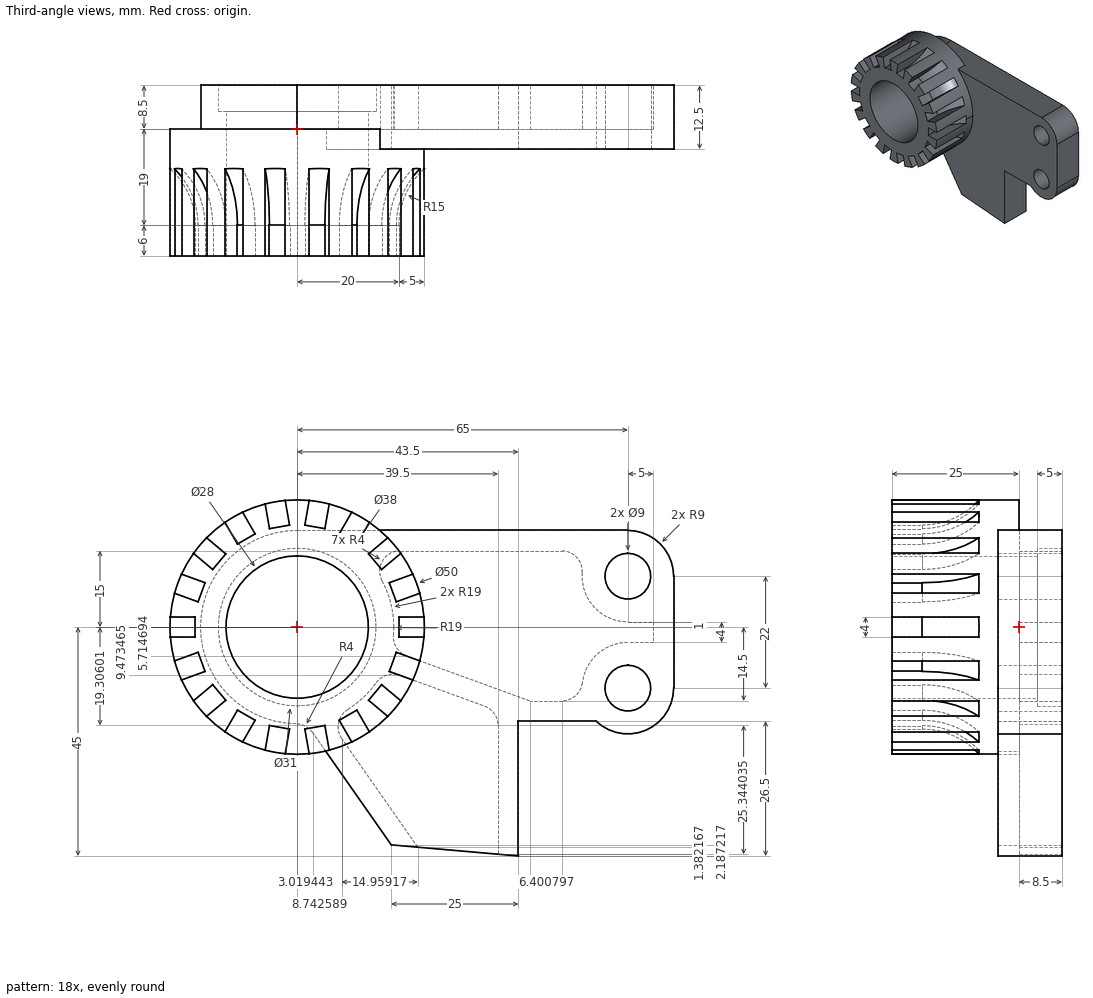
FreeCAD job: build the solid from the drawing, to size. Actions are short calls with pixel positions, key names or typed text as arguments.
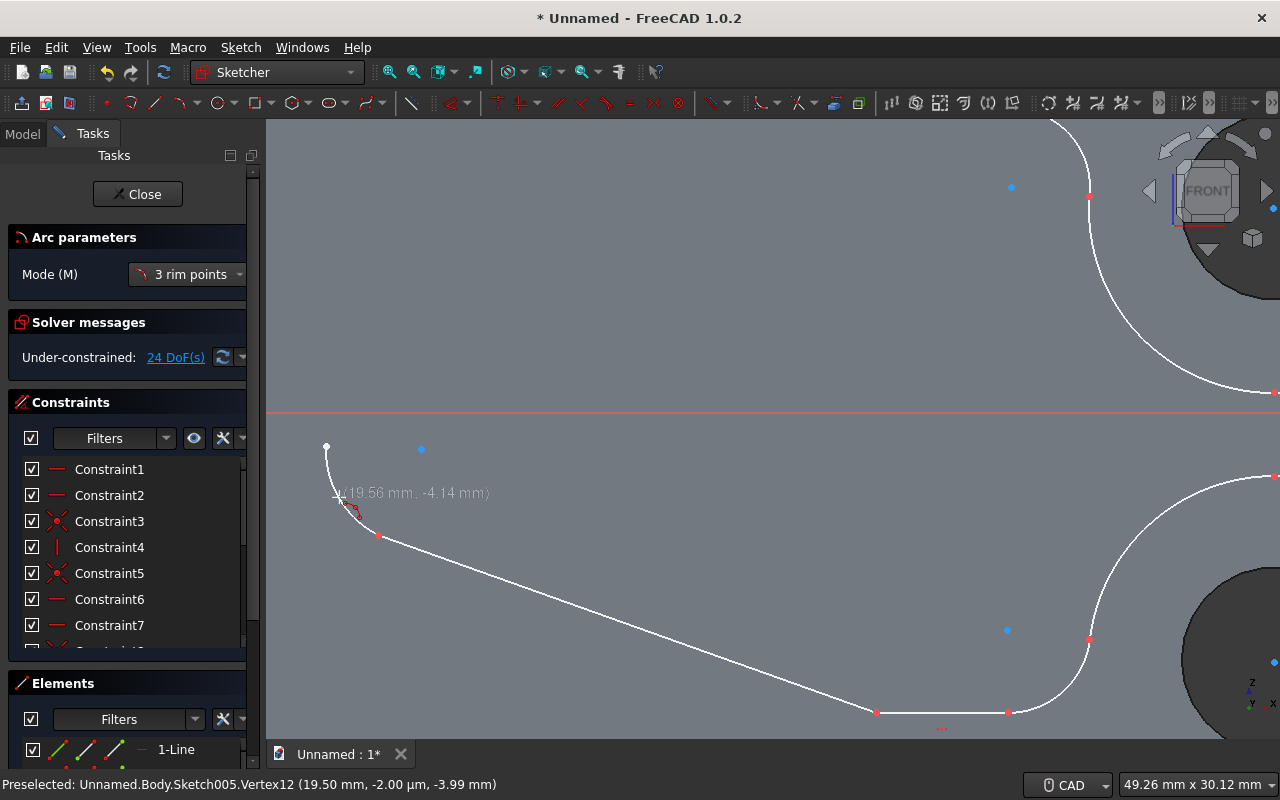
click(326, 447)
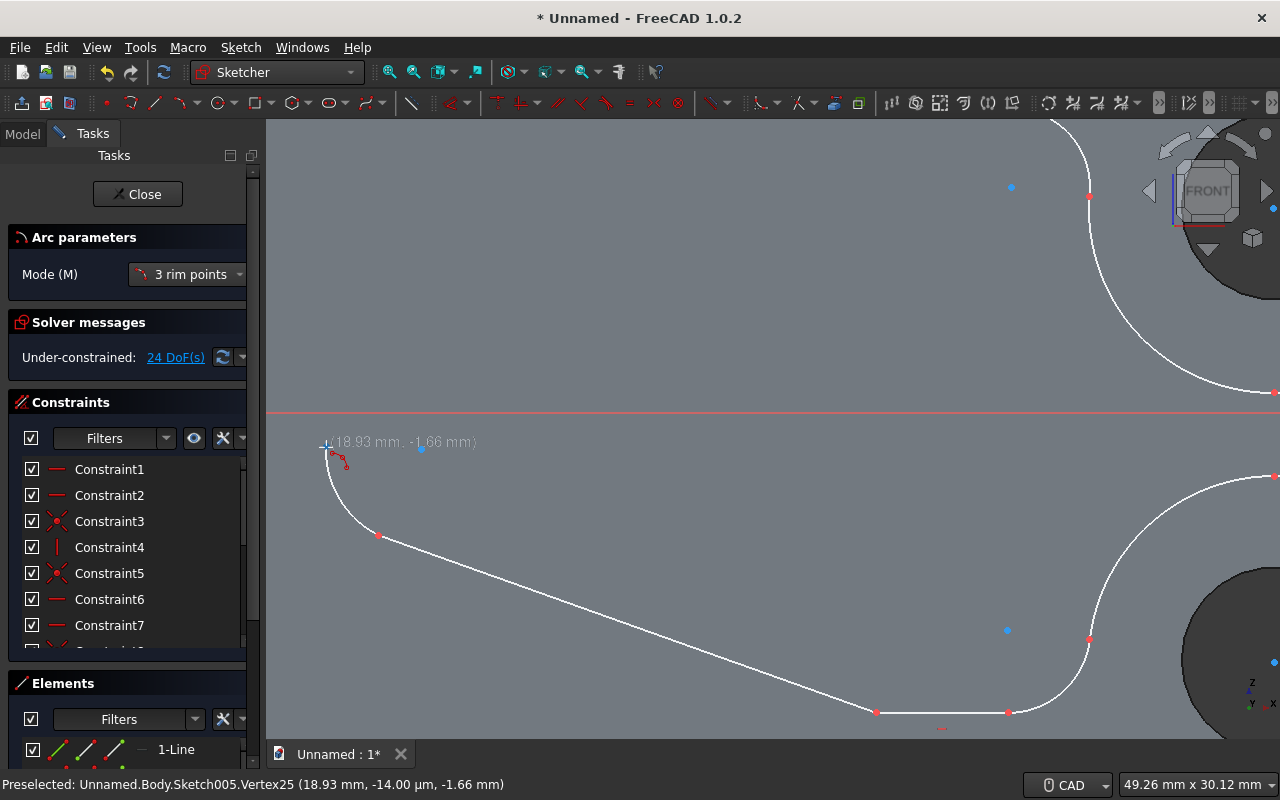
scroll(725, 304, down, 6)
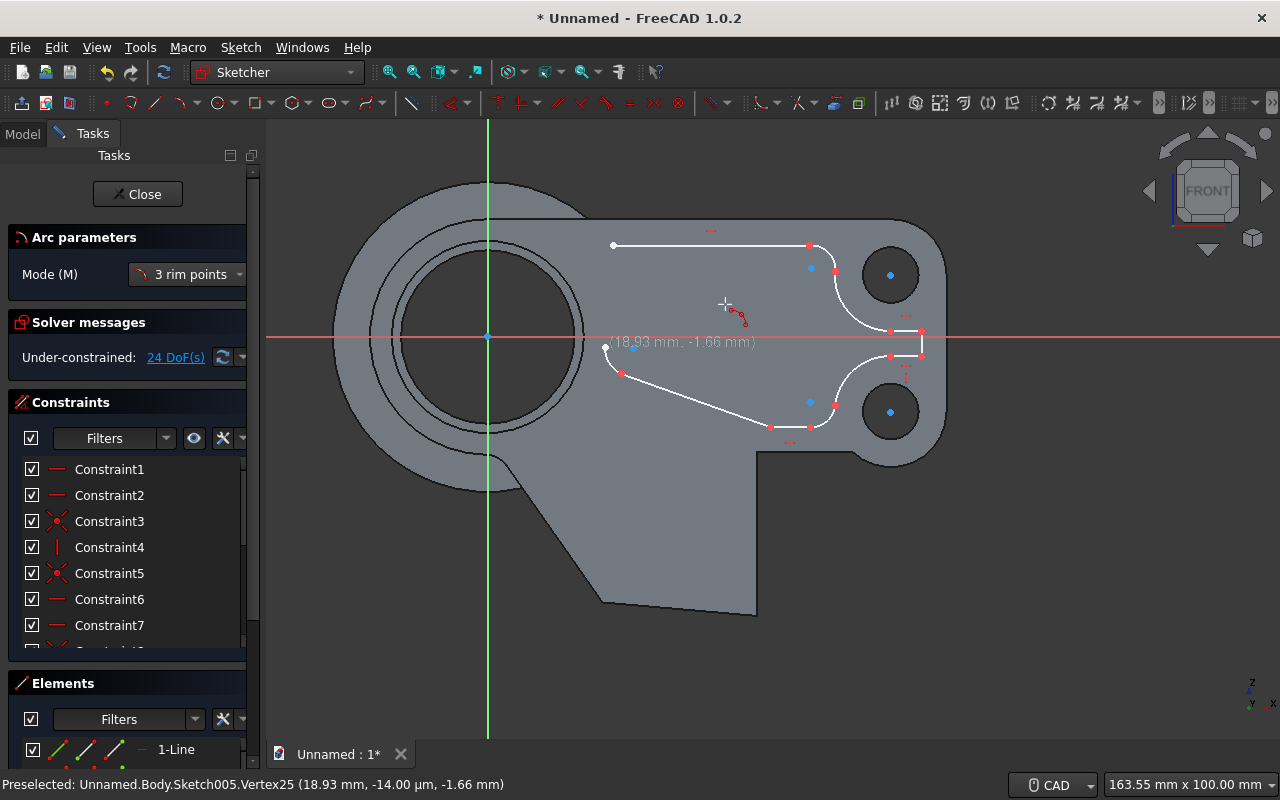
click(591, 281)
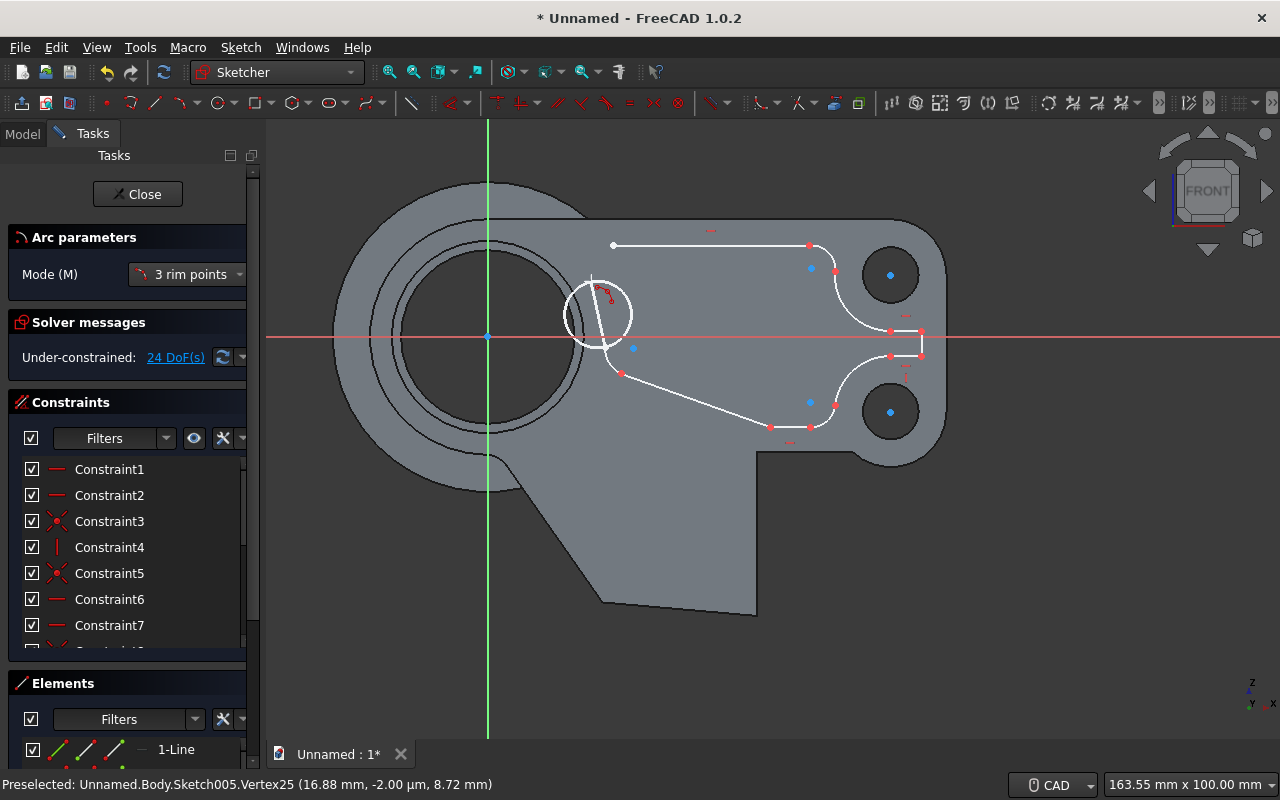
scroll(603, 313, up, 6)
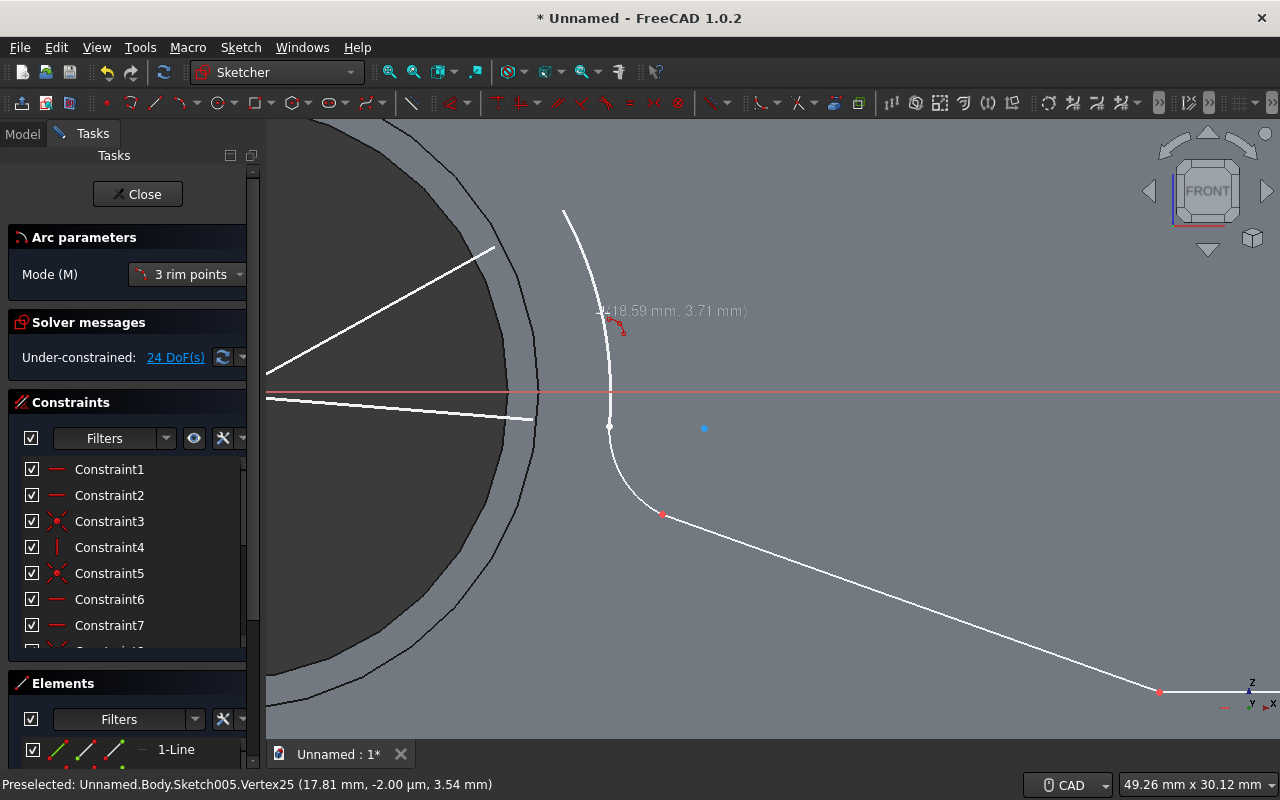
click(602, 312)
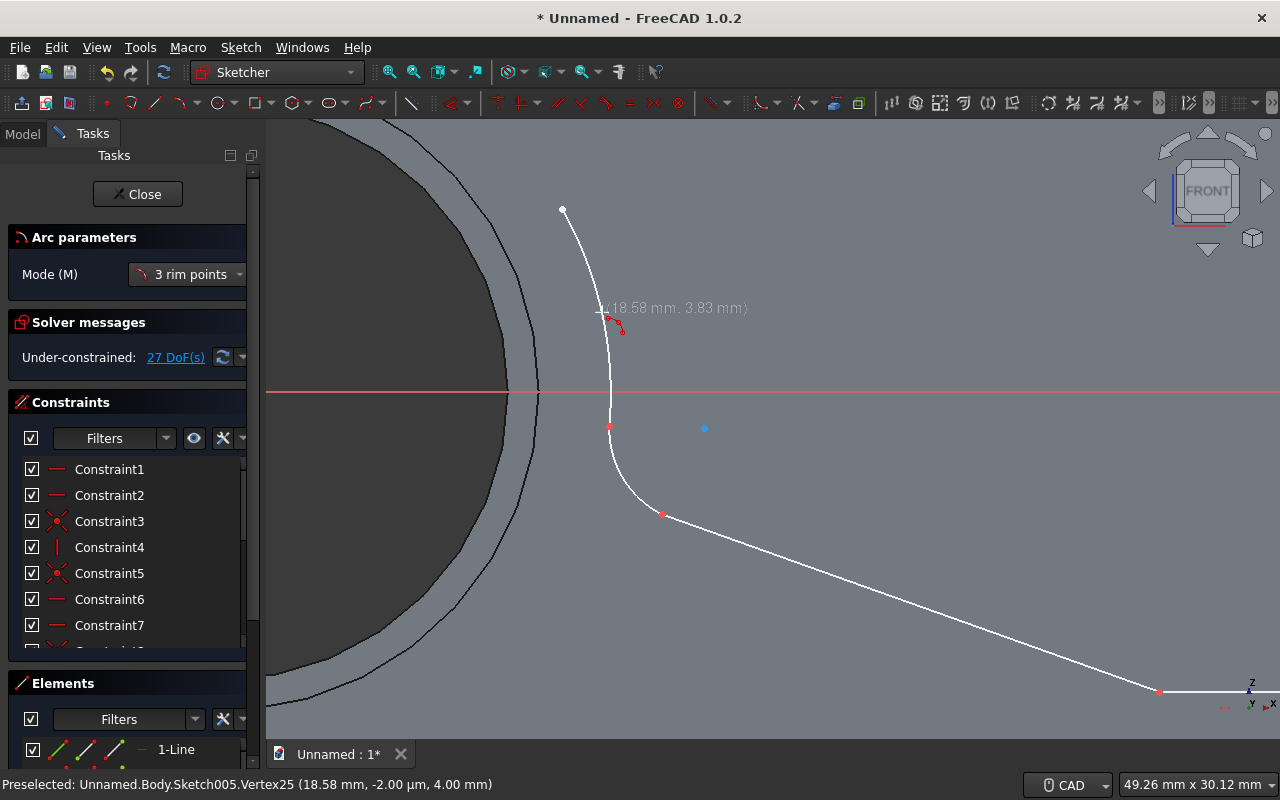
scroll(603, 313, down, 6)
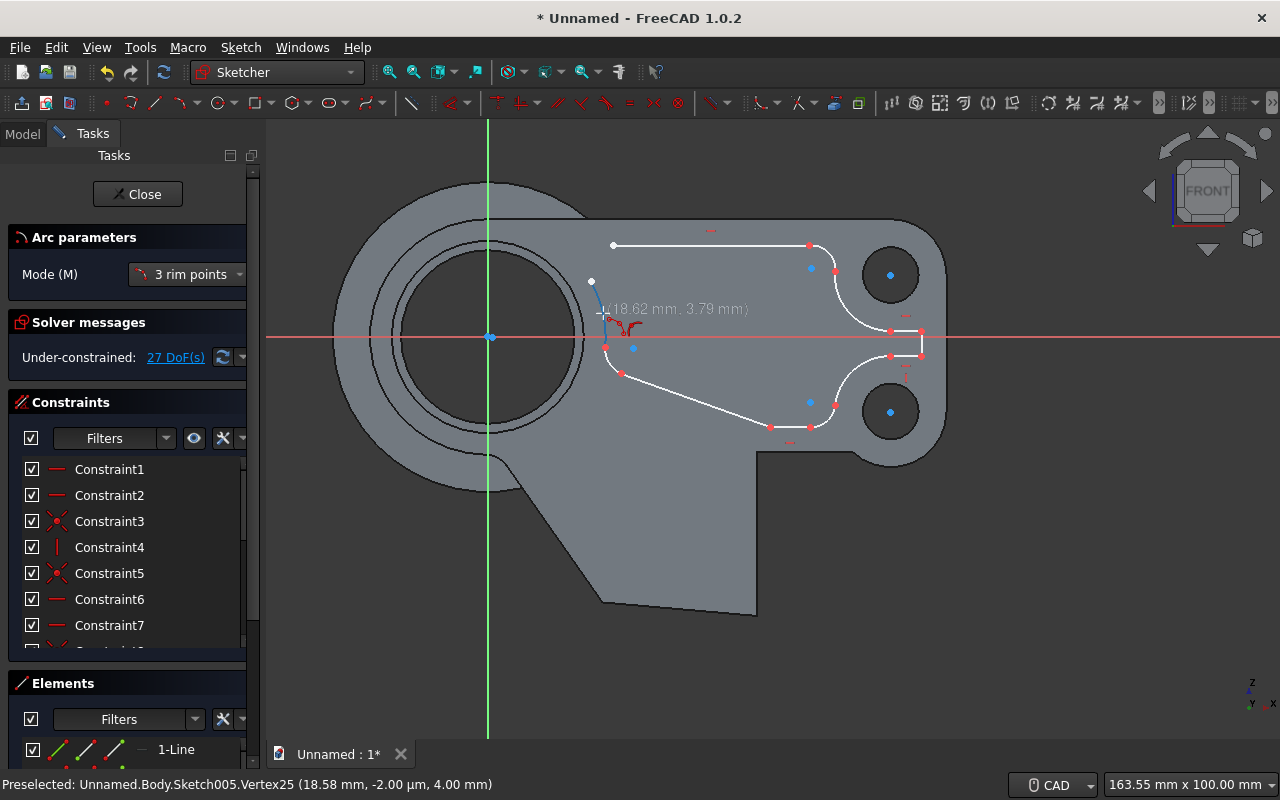
click(591, 282)
click(613, 246)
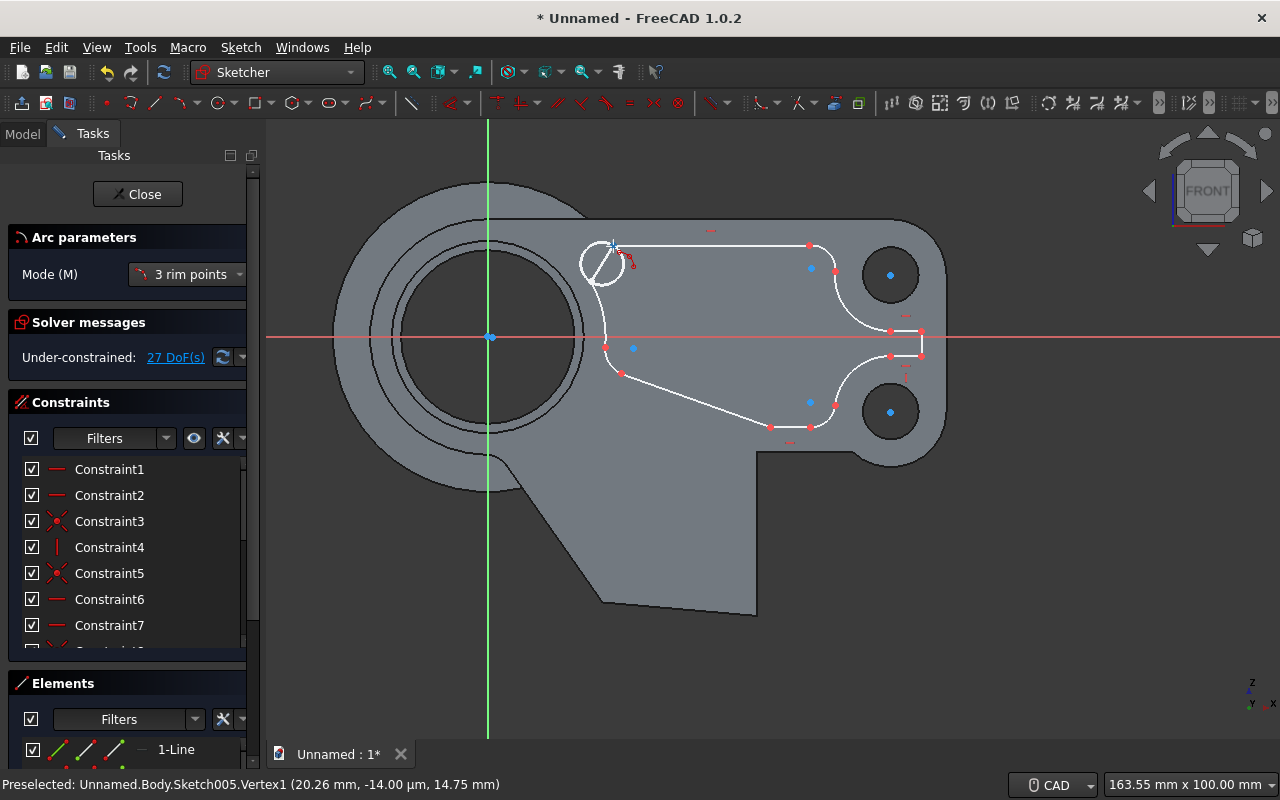
scroll(592, 256, up, 2)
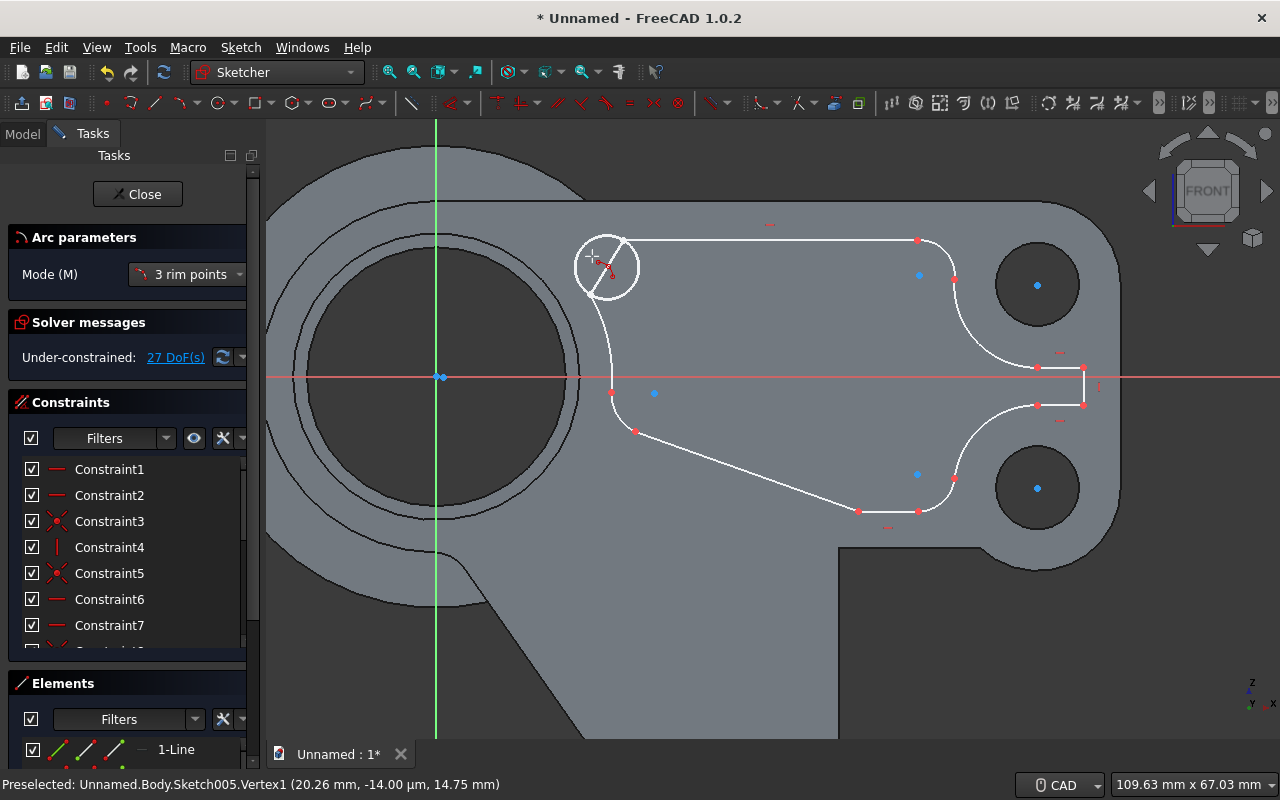
click(591, 256)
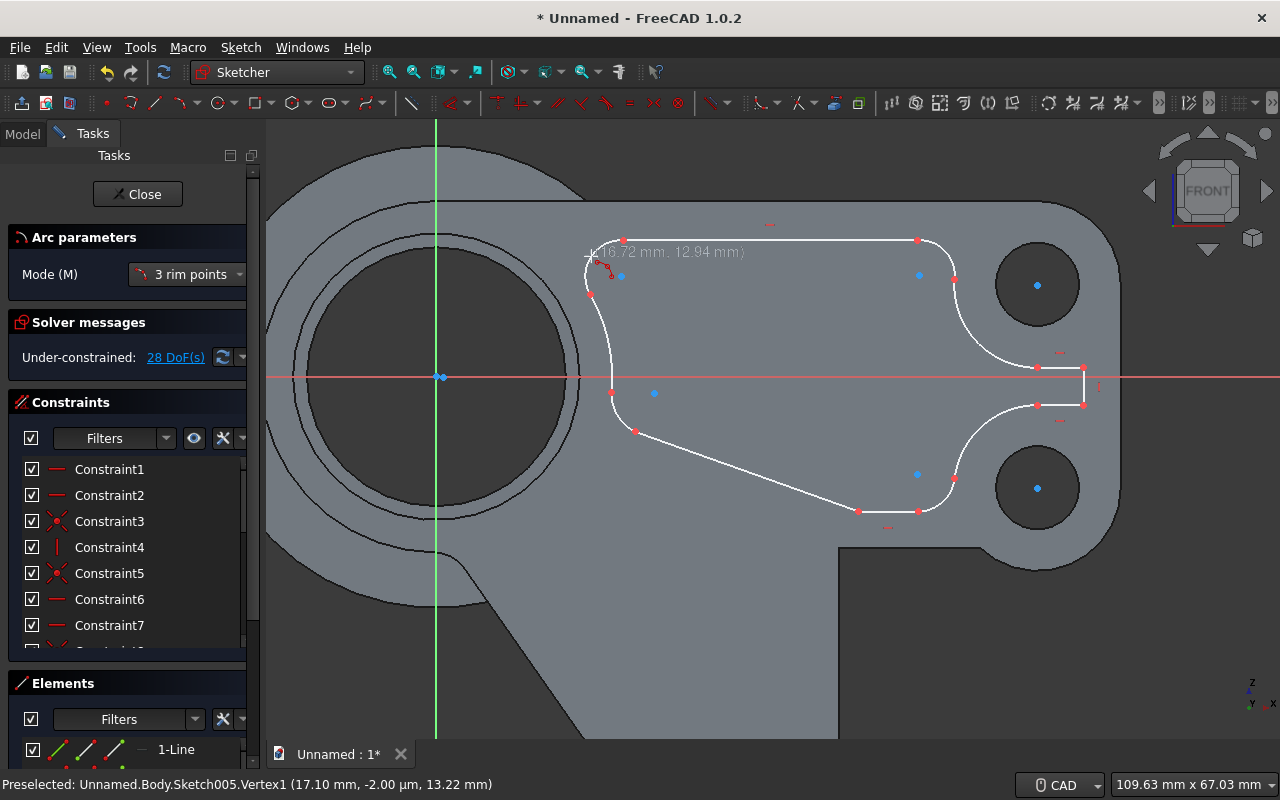
click(156, 104)